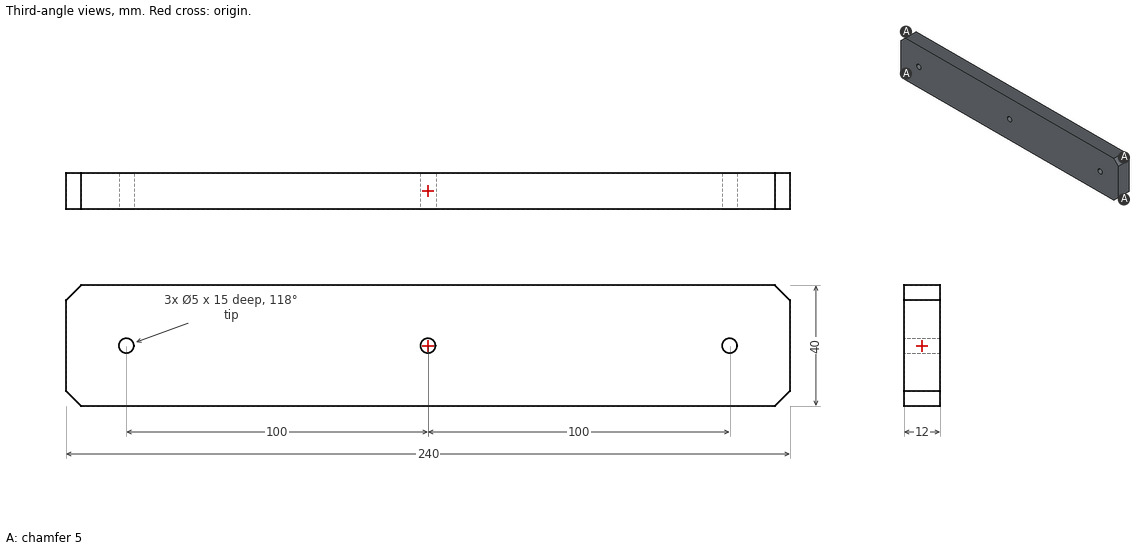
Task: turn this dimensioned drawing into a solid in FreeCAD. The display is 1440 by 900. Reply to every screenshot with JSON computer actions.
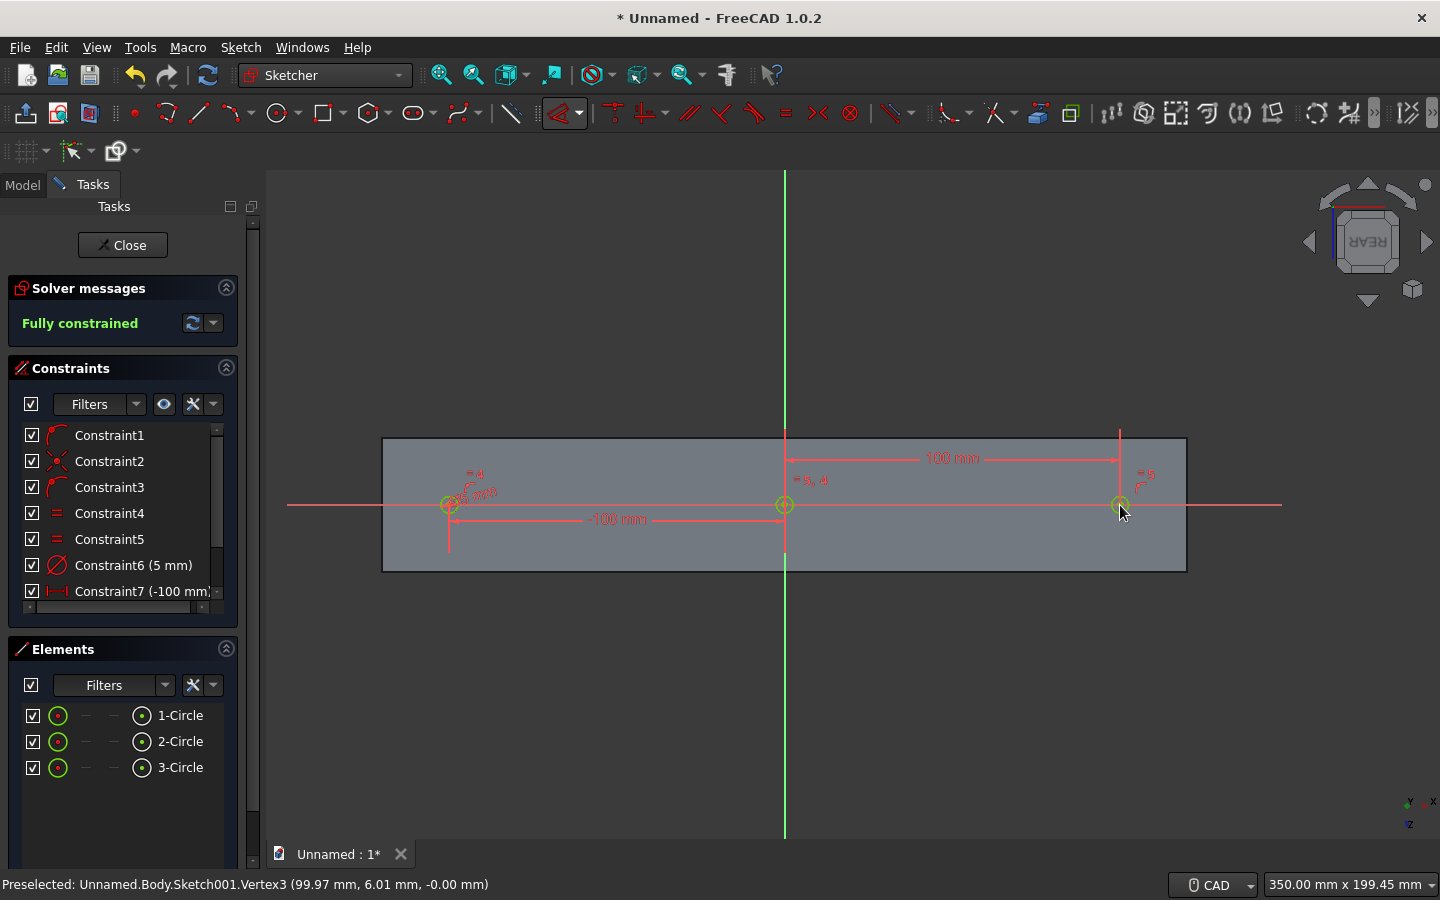
{"action": "left_click", "coordinate": [123, 245]}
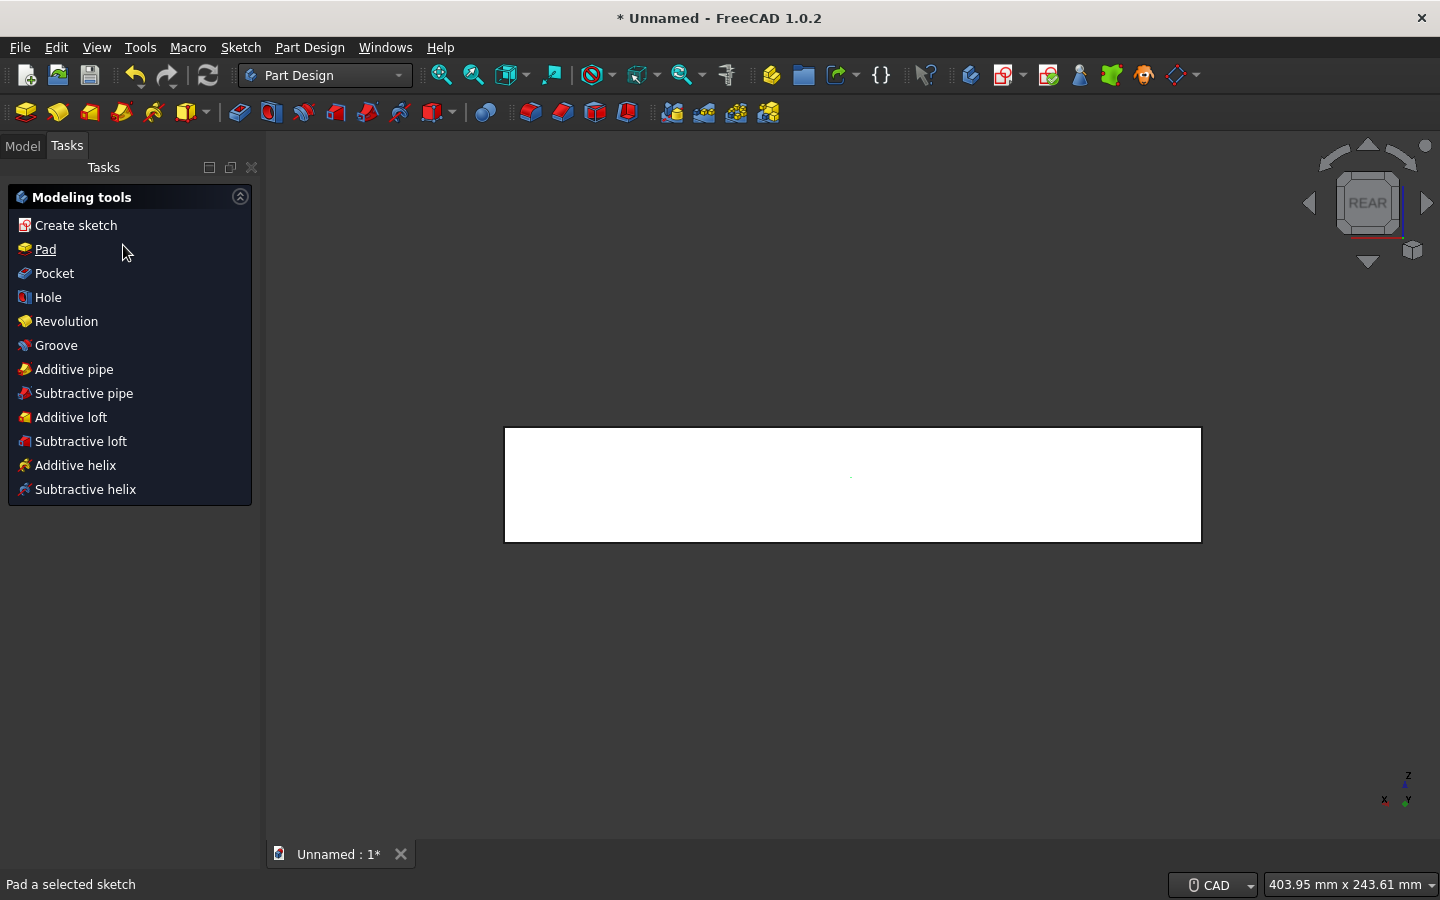
{"action": "left_click", "coordinate": [272, 112]}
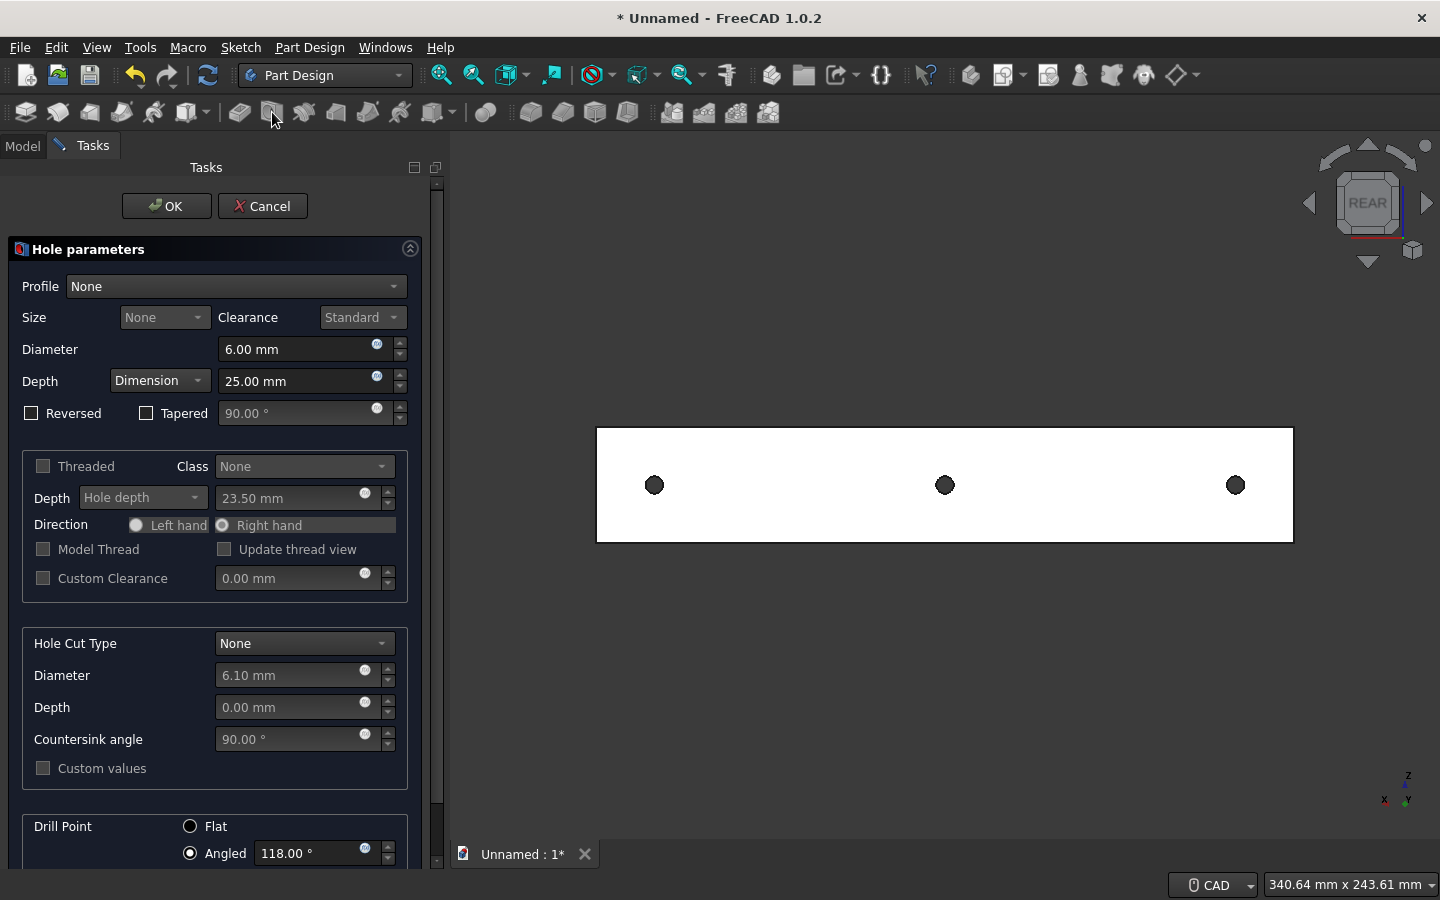
{"action": "triple_click", "coordinate": [305, 349]}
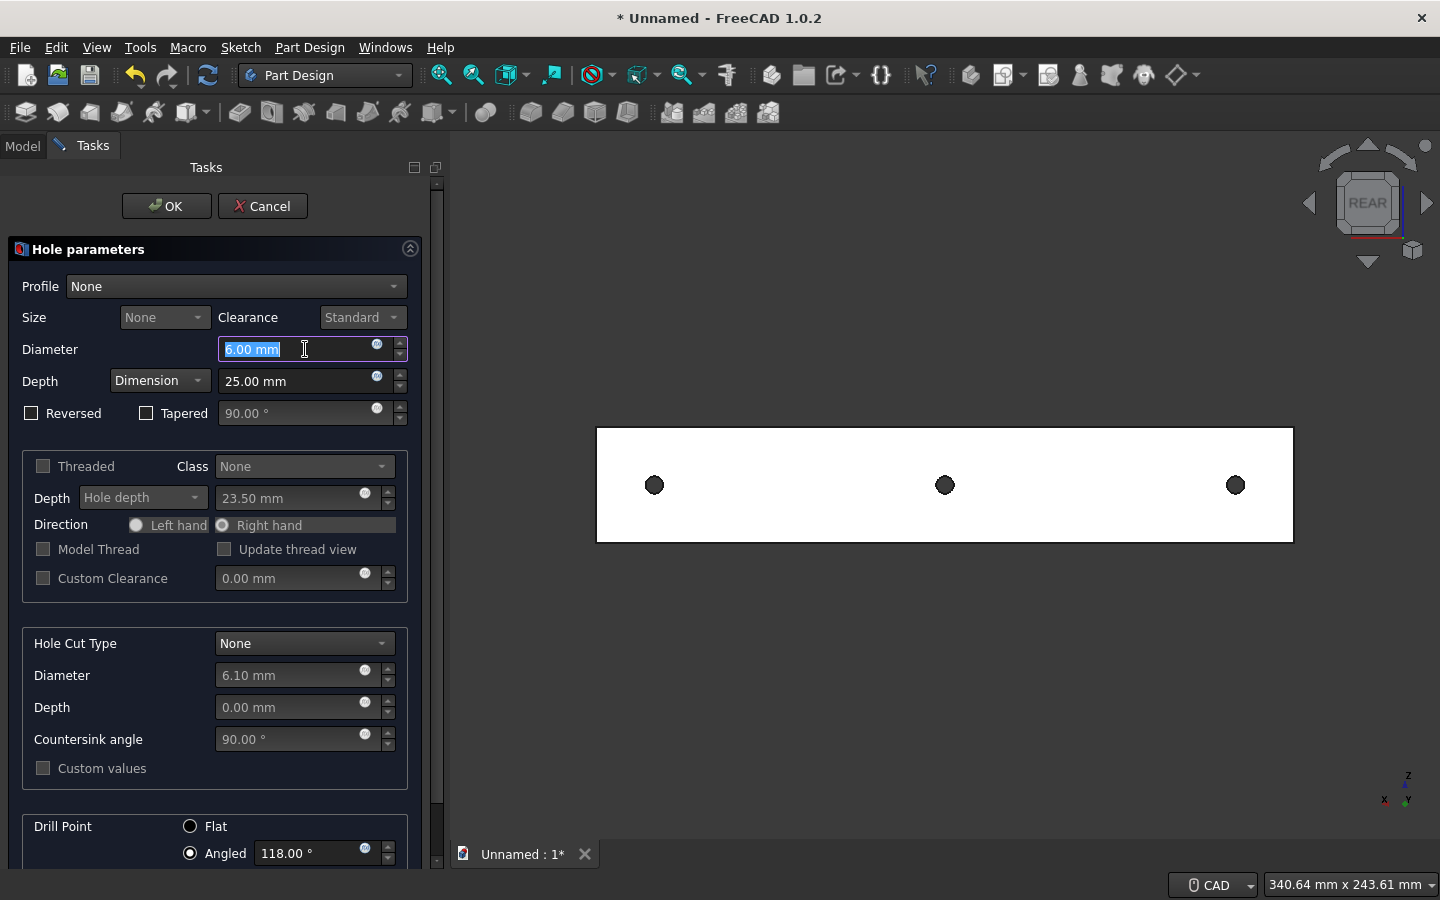
{"action": "type", "text": "5"}
{"action": "key", "text": "Tab"}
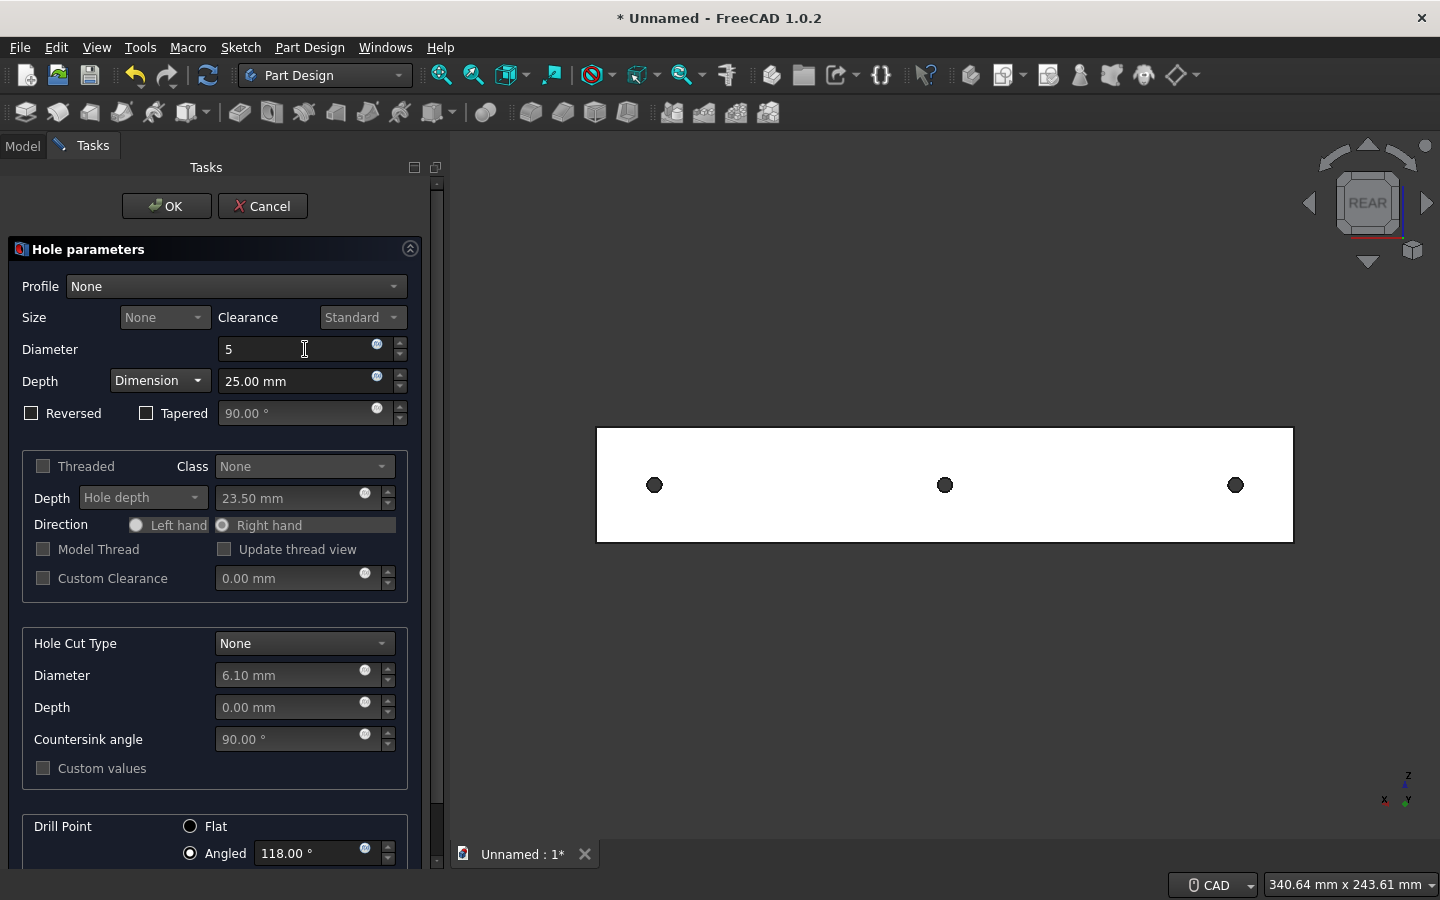
{"action": "triple_click", "coordinate": [305, 381]}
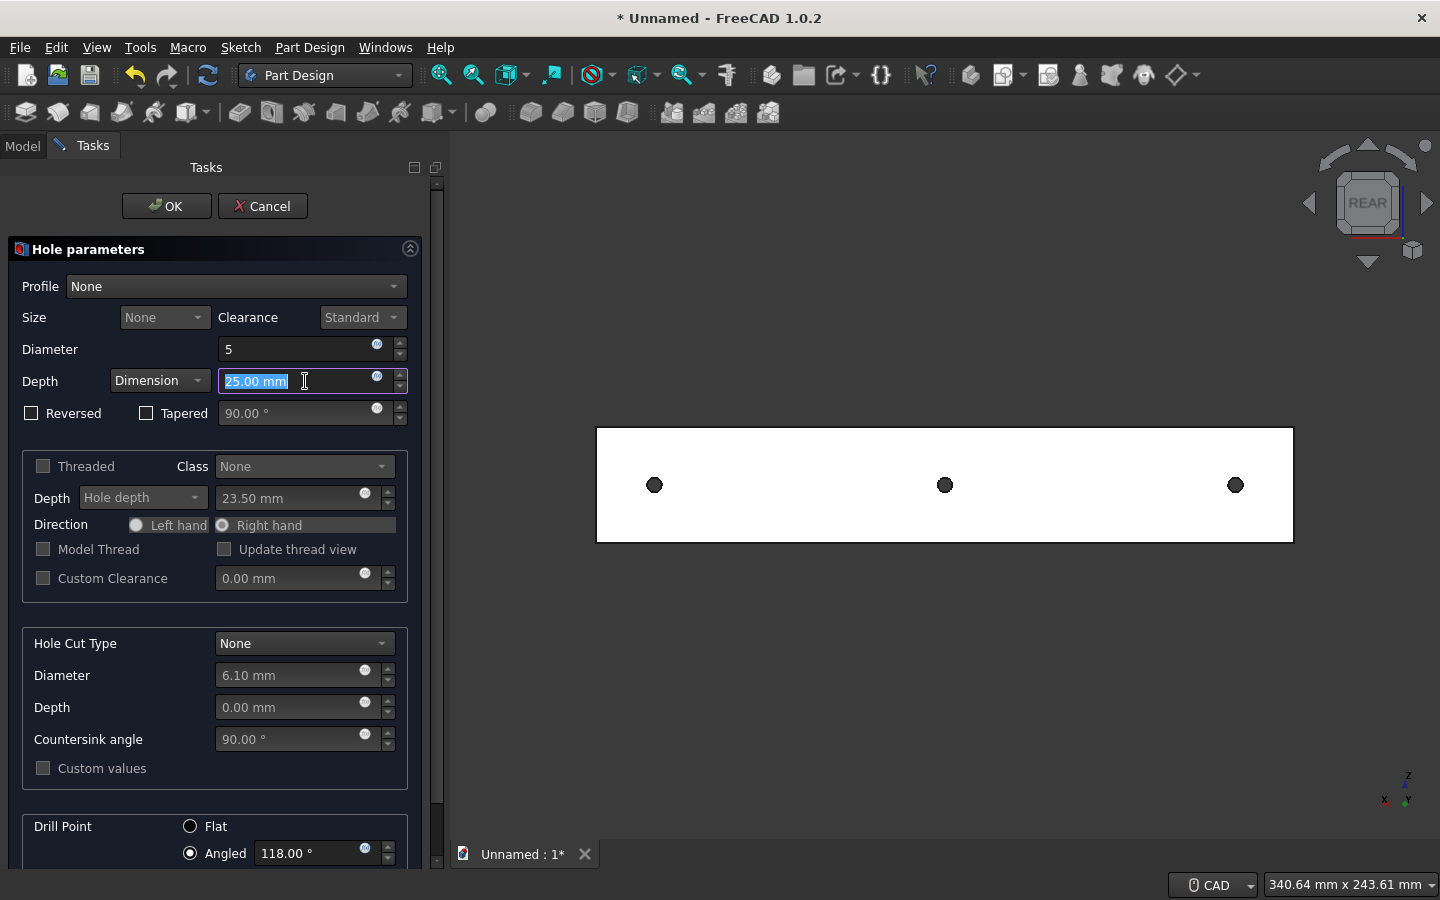
{"action": "type", "text": "15"}
{"action": "key", "text": "Tab"}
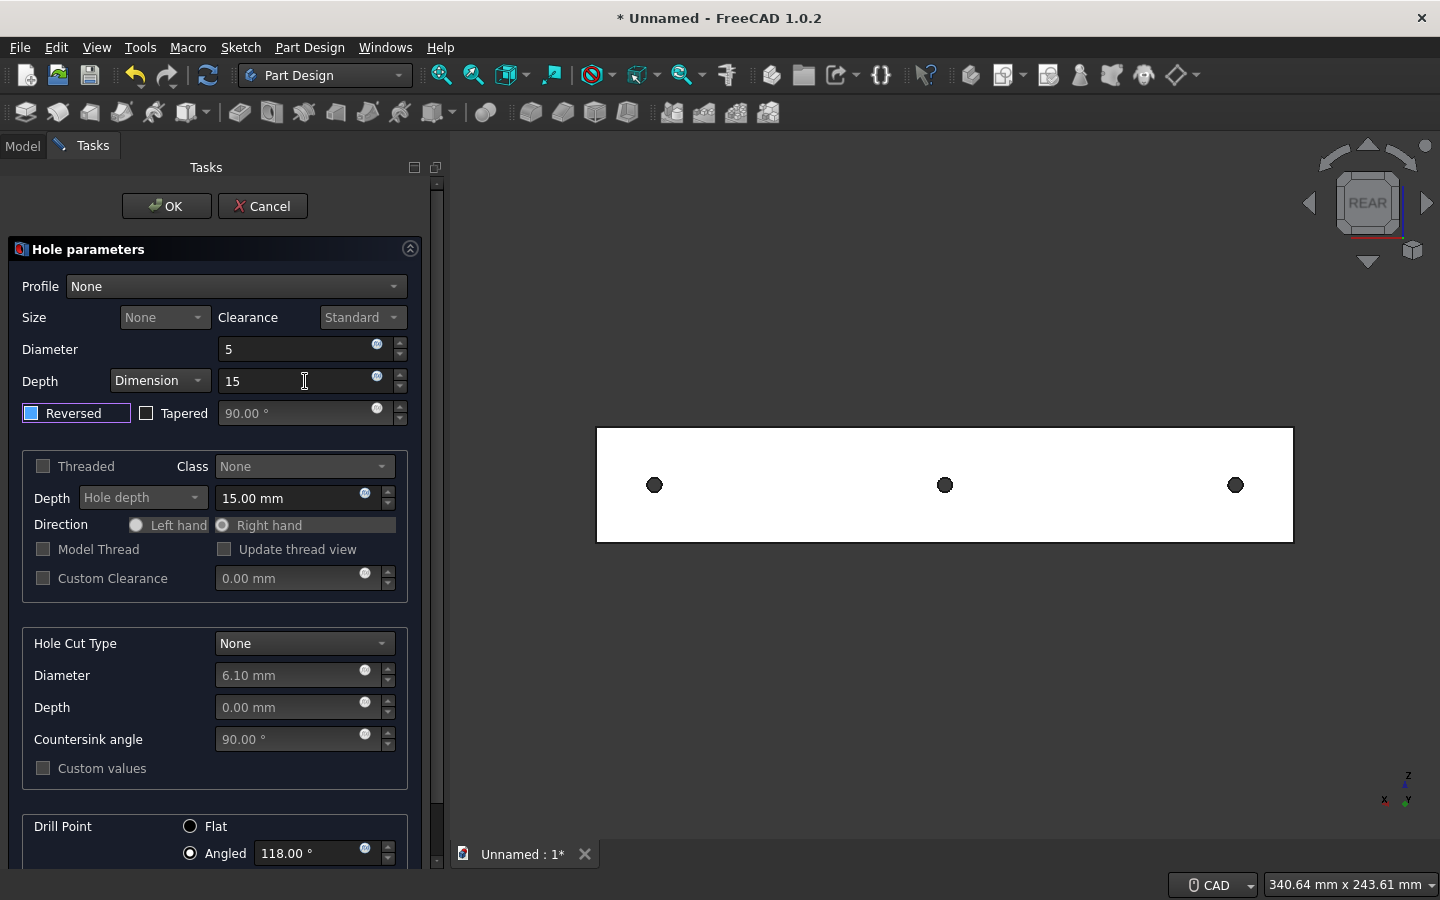
{"action": "left_click", "coordinate": [167, 206]}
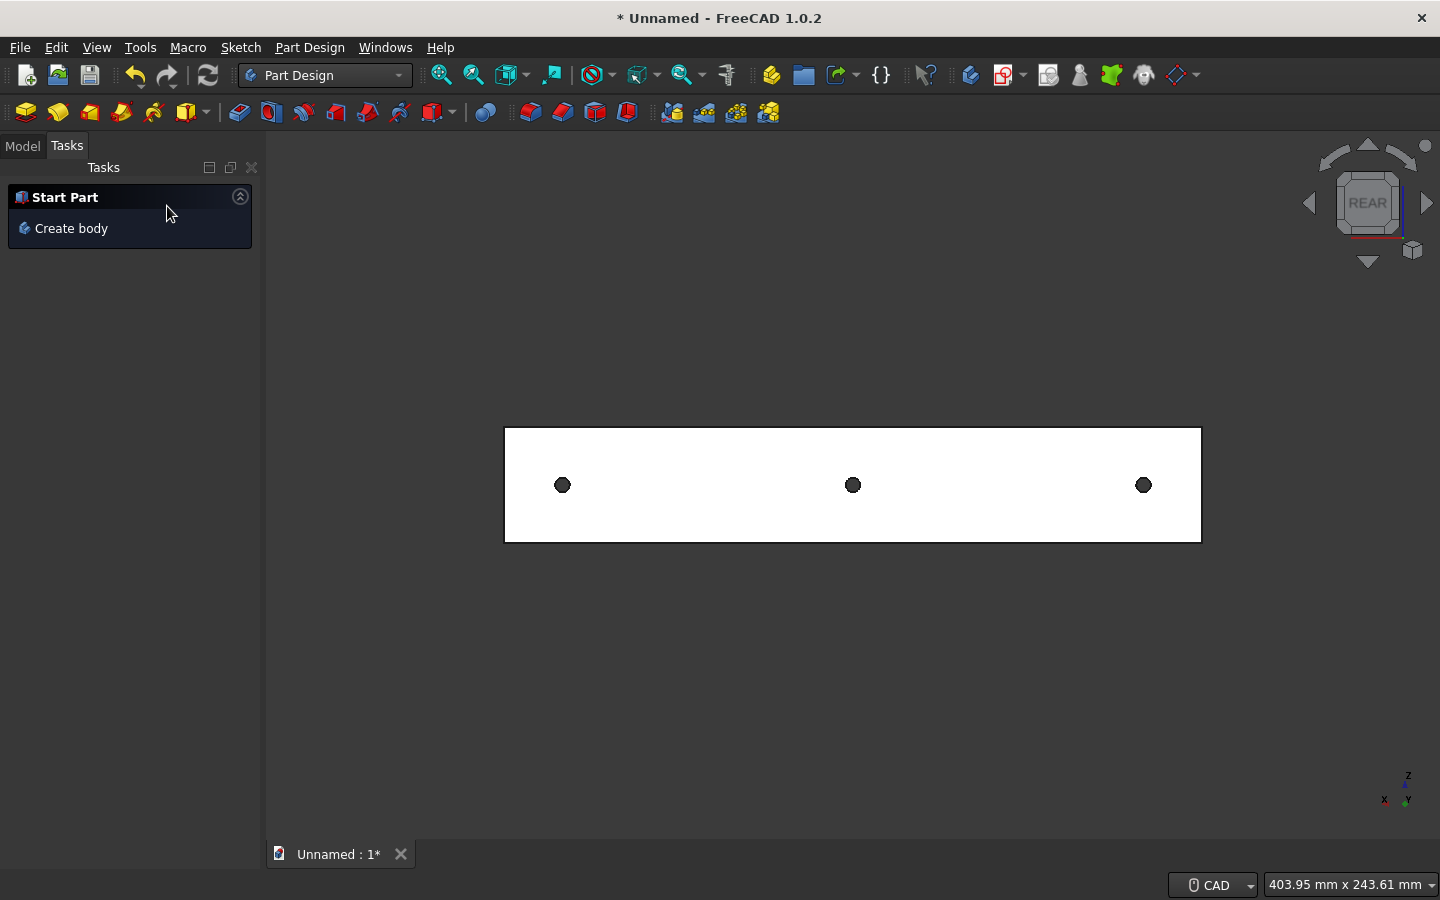
{"action": "key", "text": "0"}